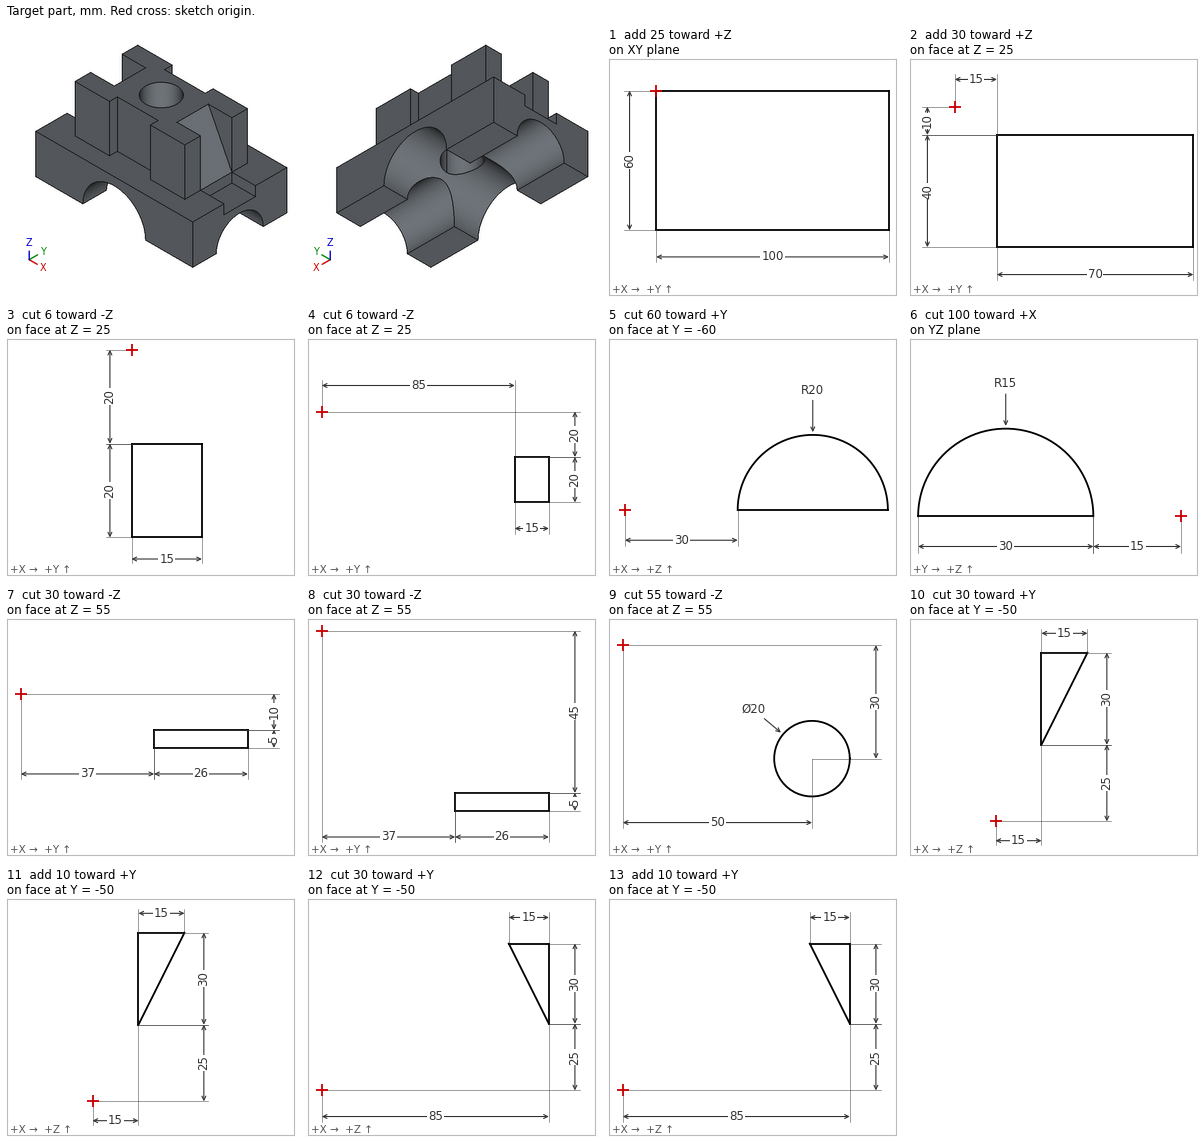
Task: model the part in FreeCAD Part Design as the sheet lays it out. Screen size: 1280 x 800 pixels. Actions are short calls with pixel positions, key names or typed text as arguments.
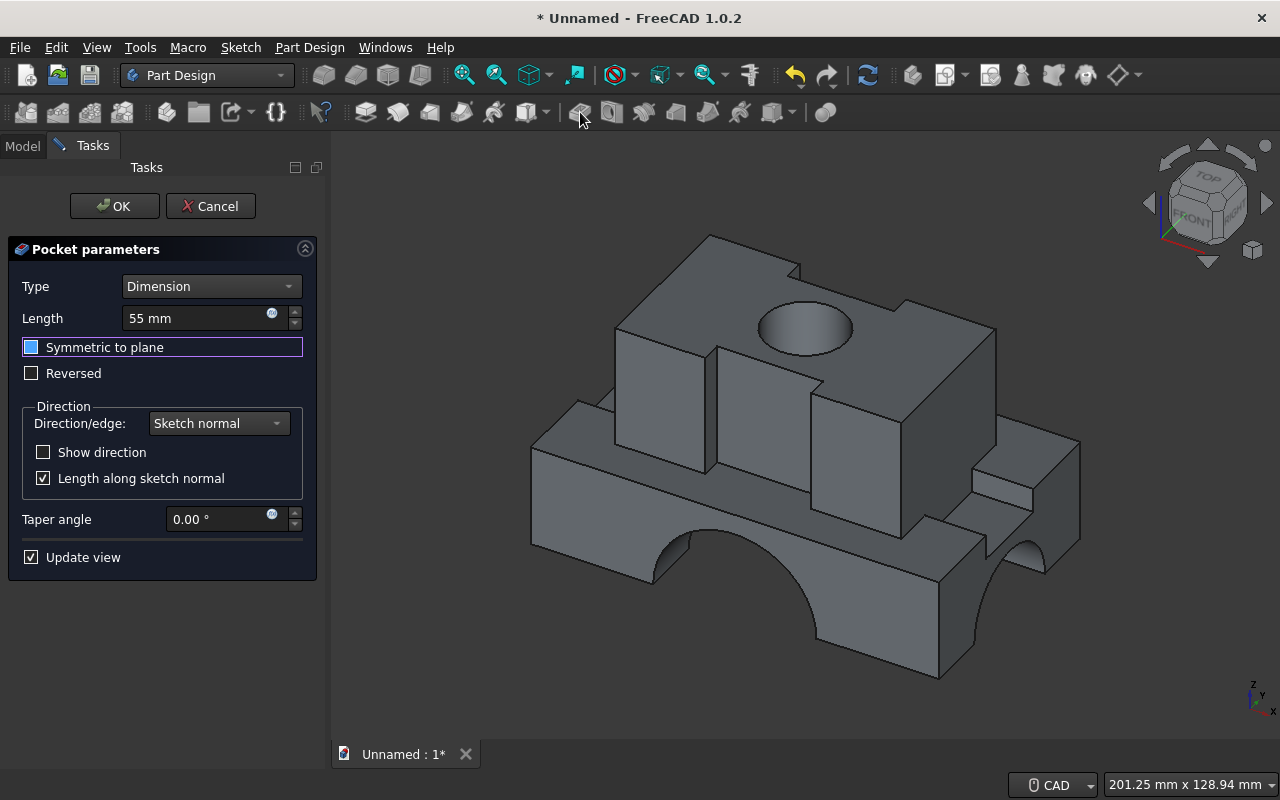
click(115, 206)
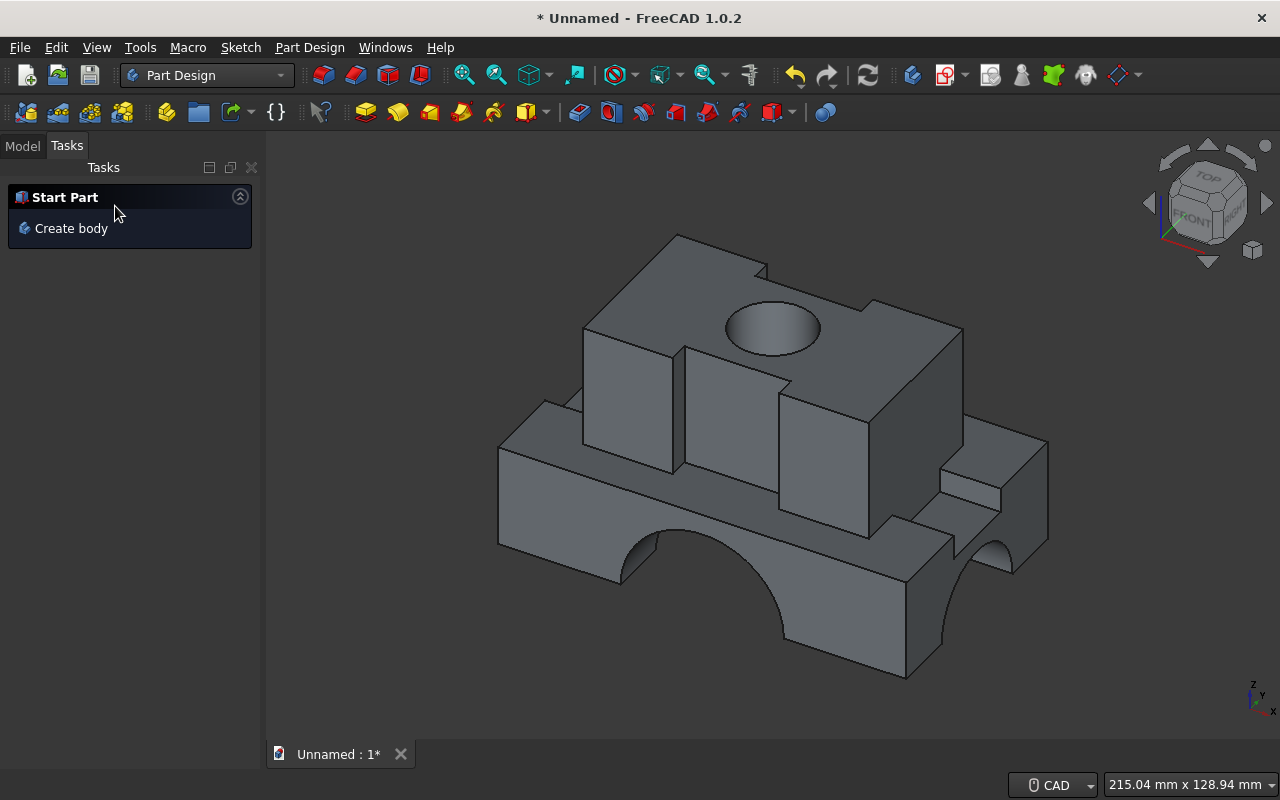
click(628, 400)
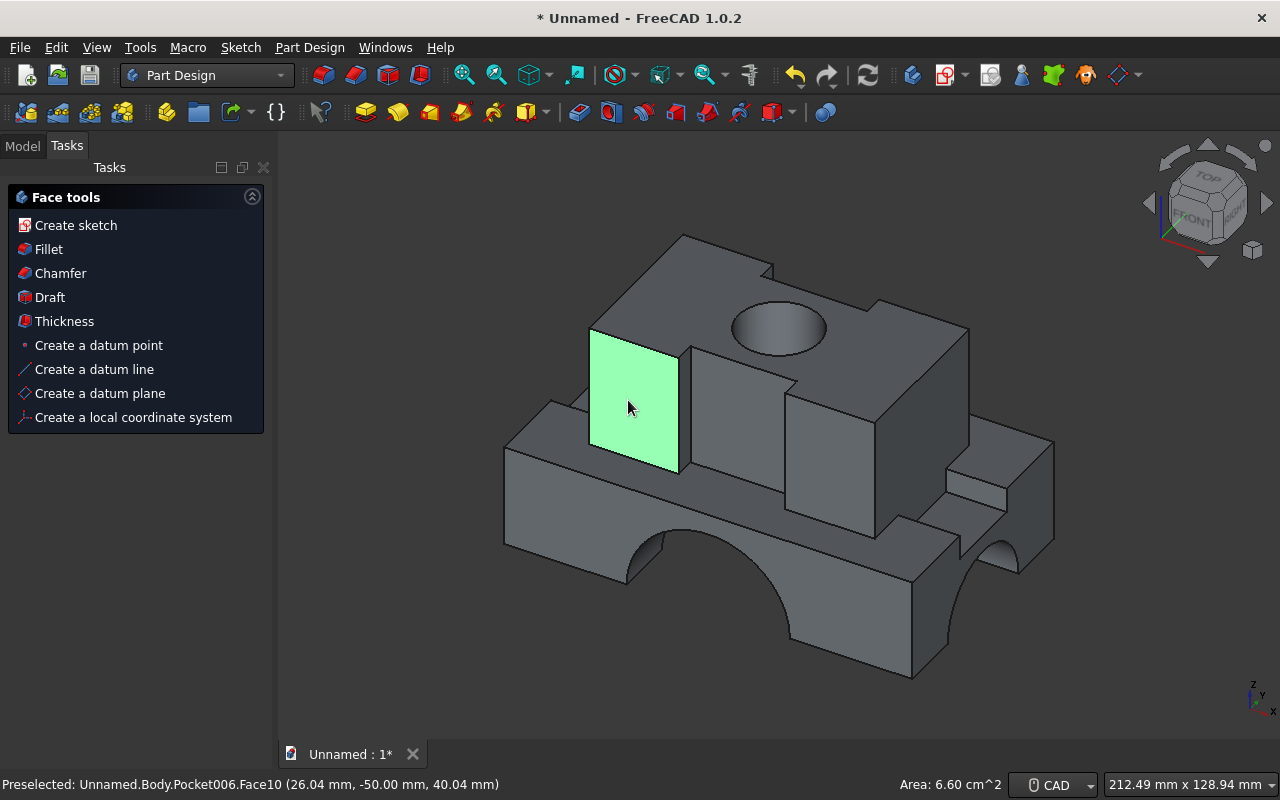
click(946, 76)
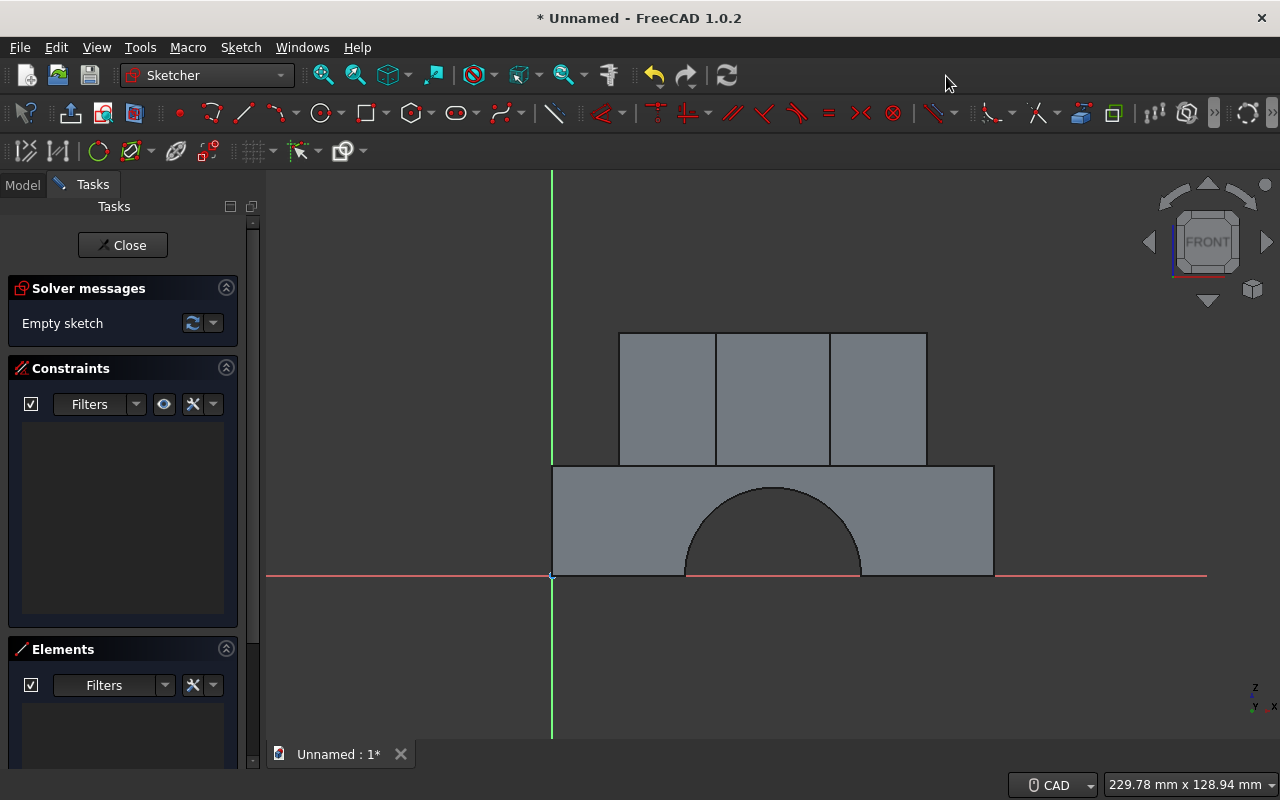
key(q)
key(s)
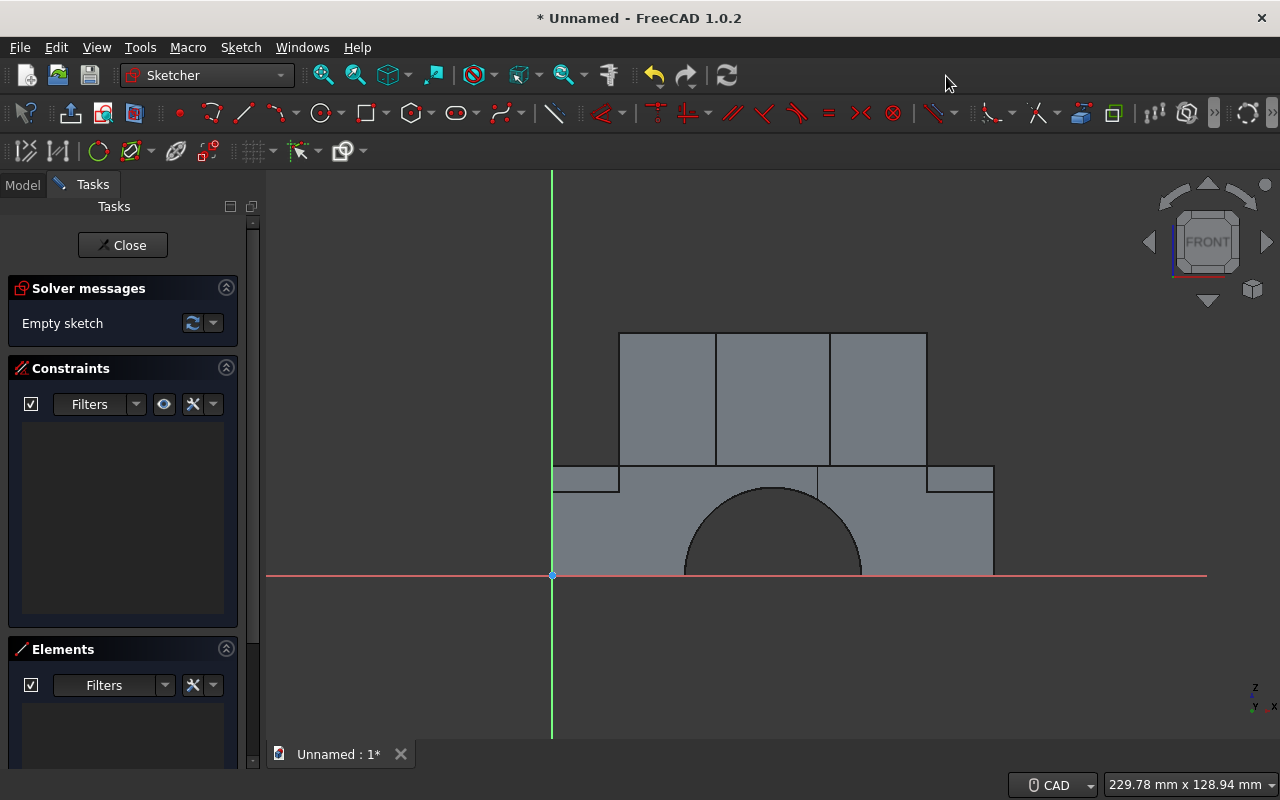
scroll(444, 454, up, 2)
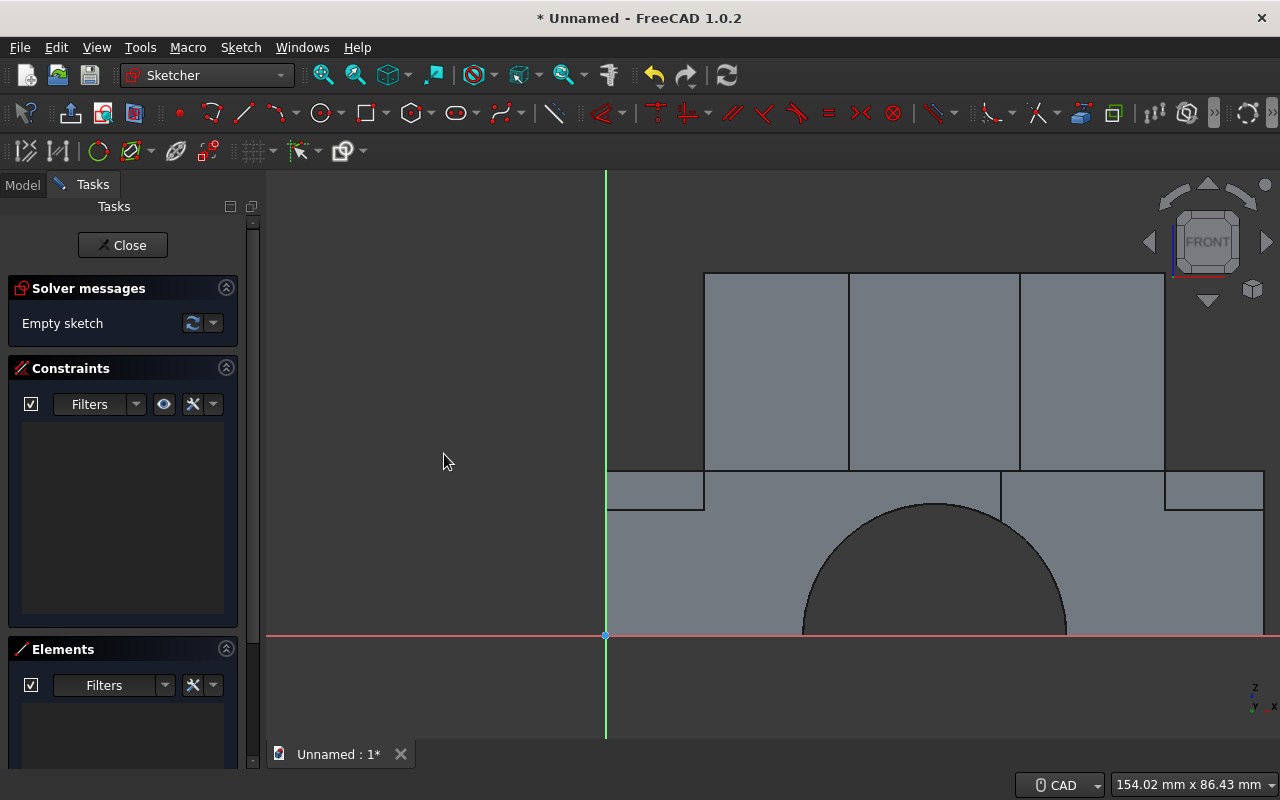
click(212, 114)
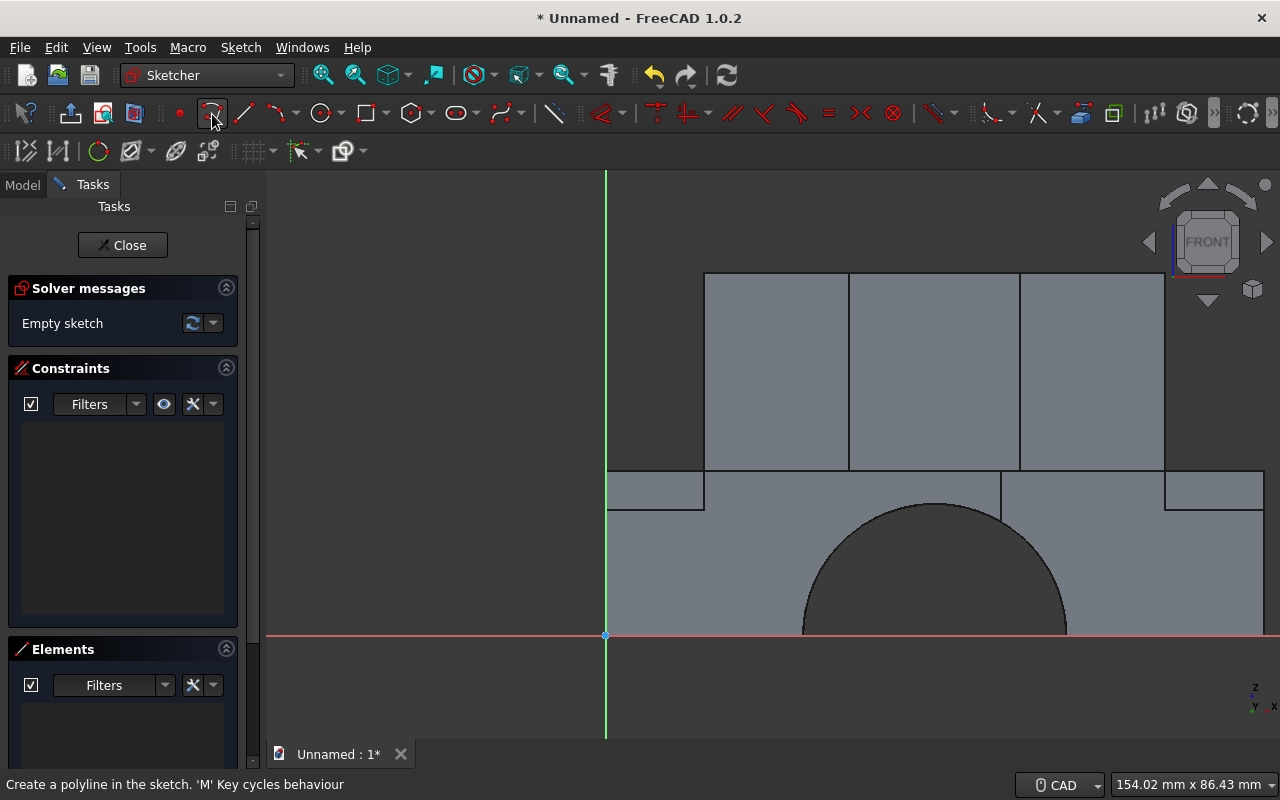
click(704, 471)
click(803, 273)
click(704, 273)
click(704, 472)
key(Escape)
key(Escape)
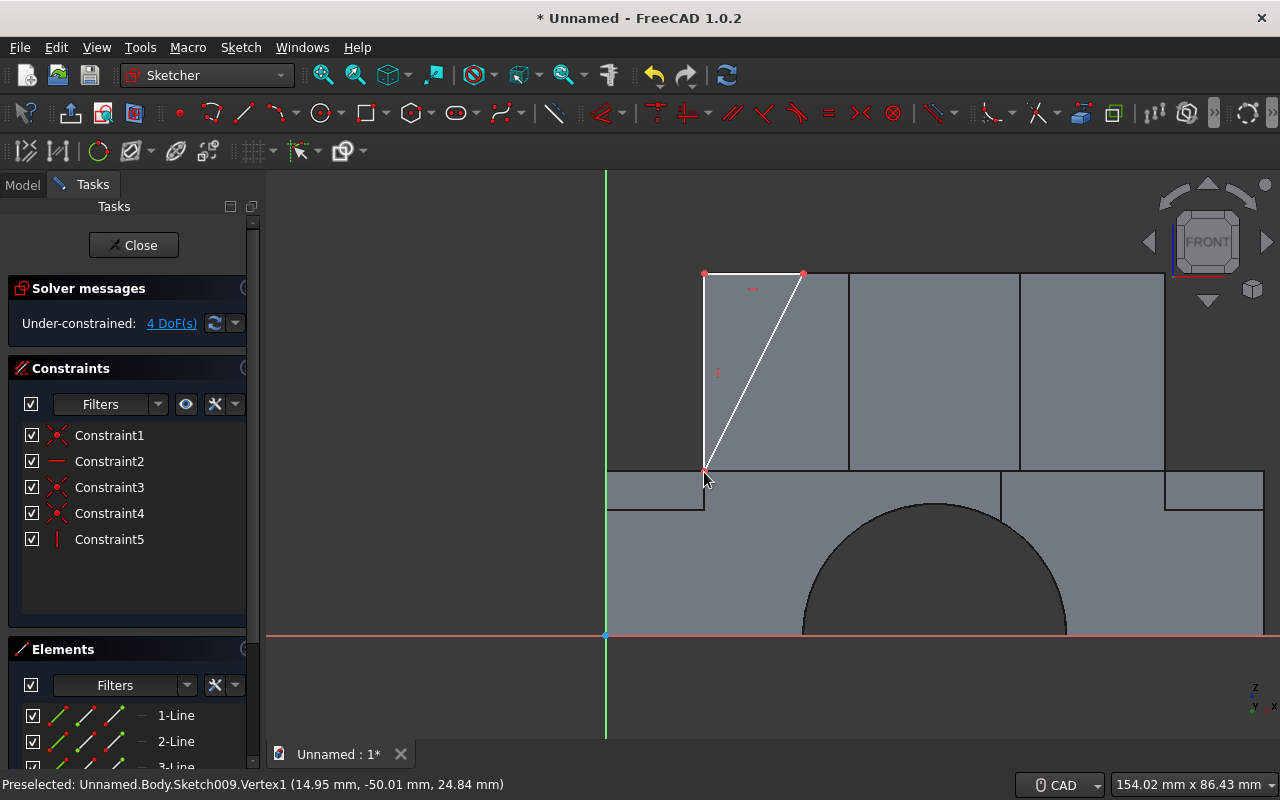
key(d)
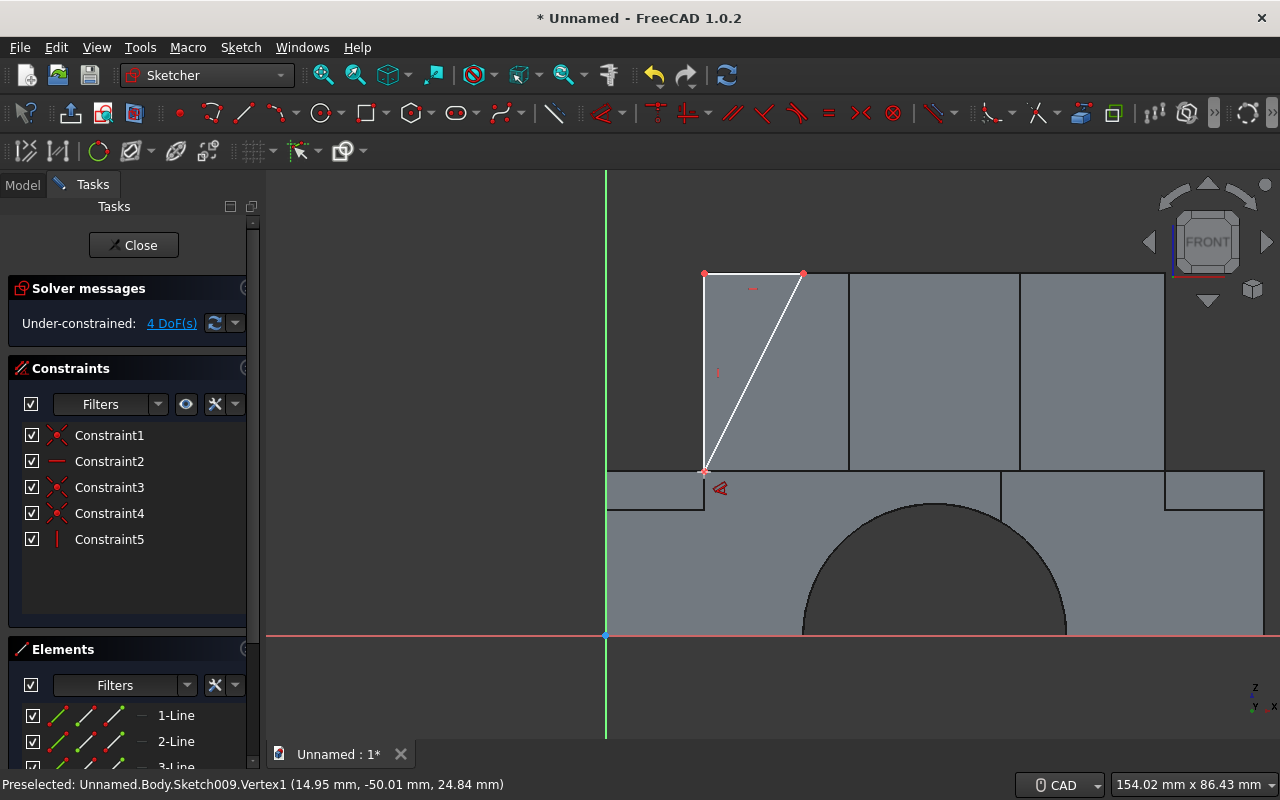
click(773, 274)
click(753, 240)